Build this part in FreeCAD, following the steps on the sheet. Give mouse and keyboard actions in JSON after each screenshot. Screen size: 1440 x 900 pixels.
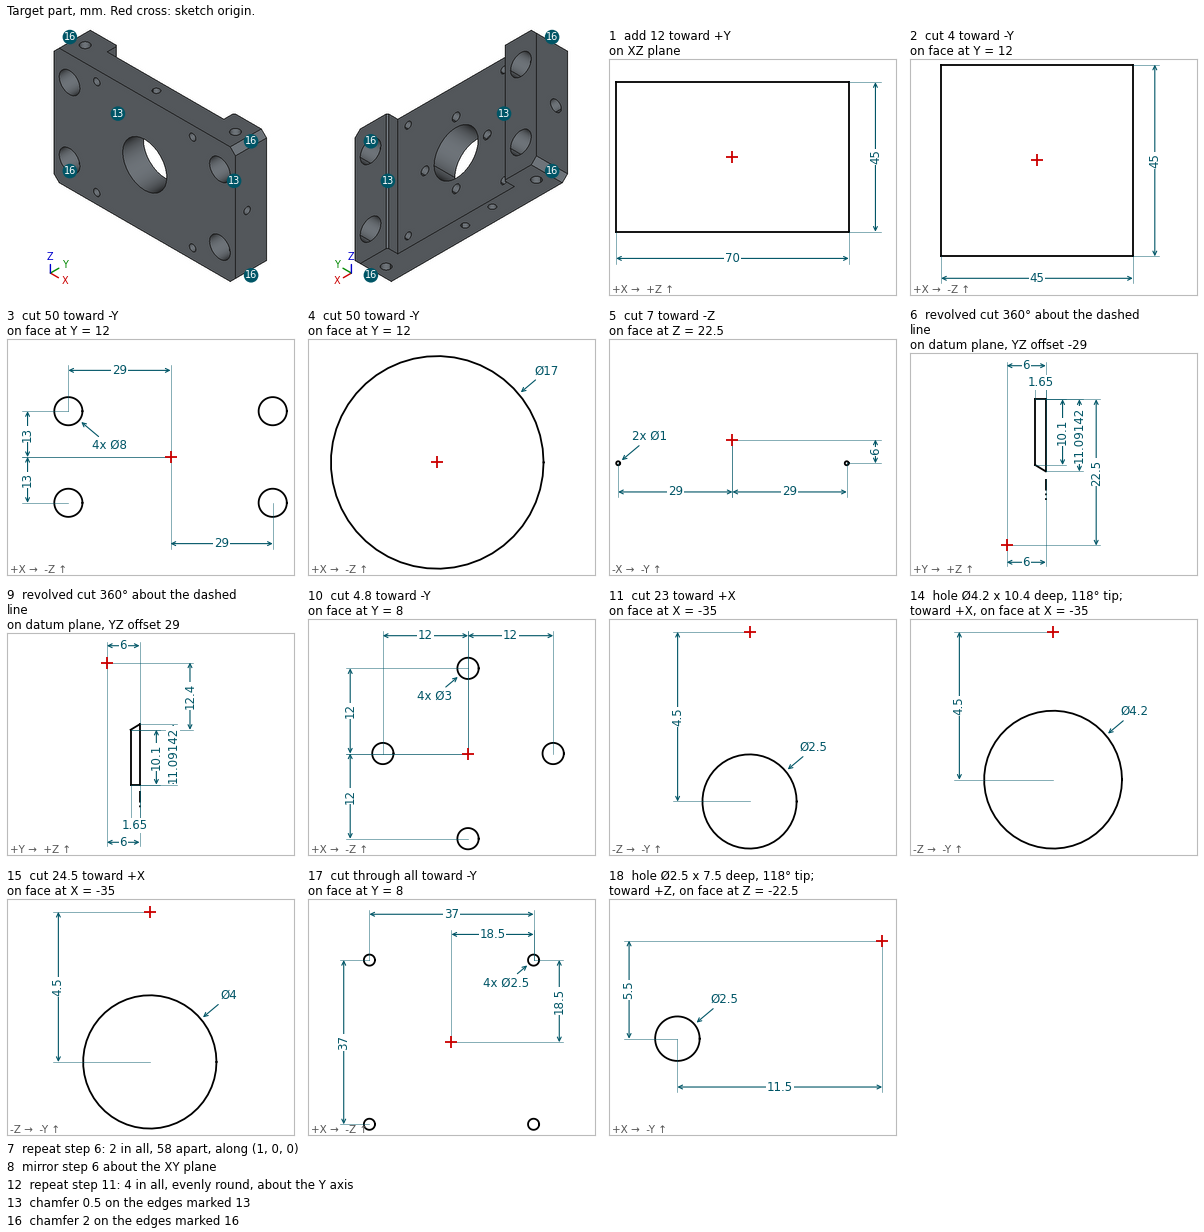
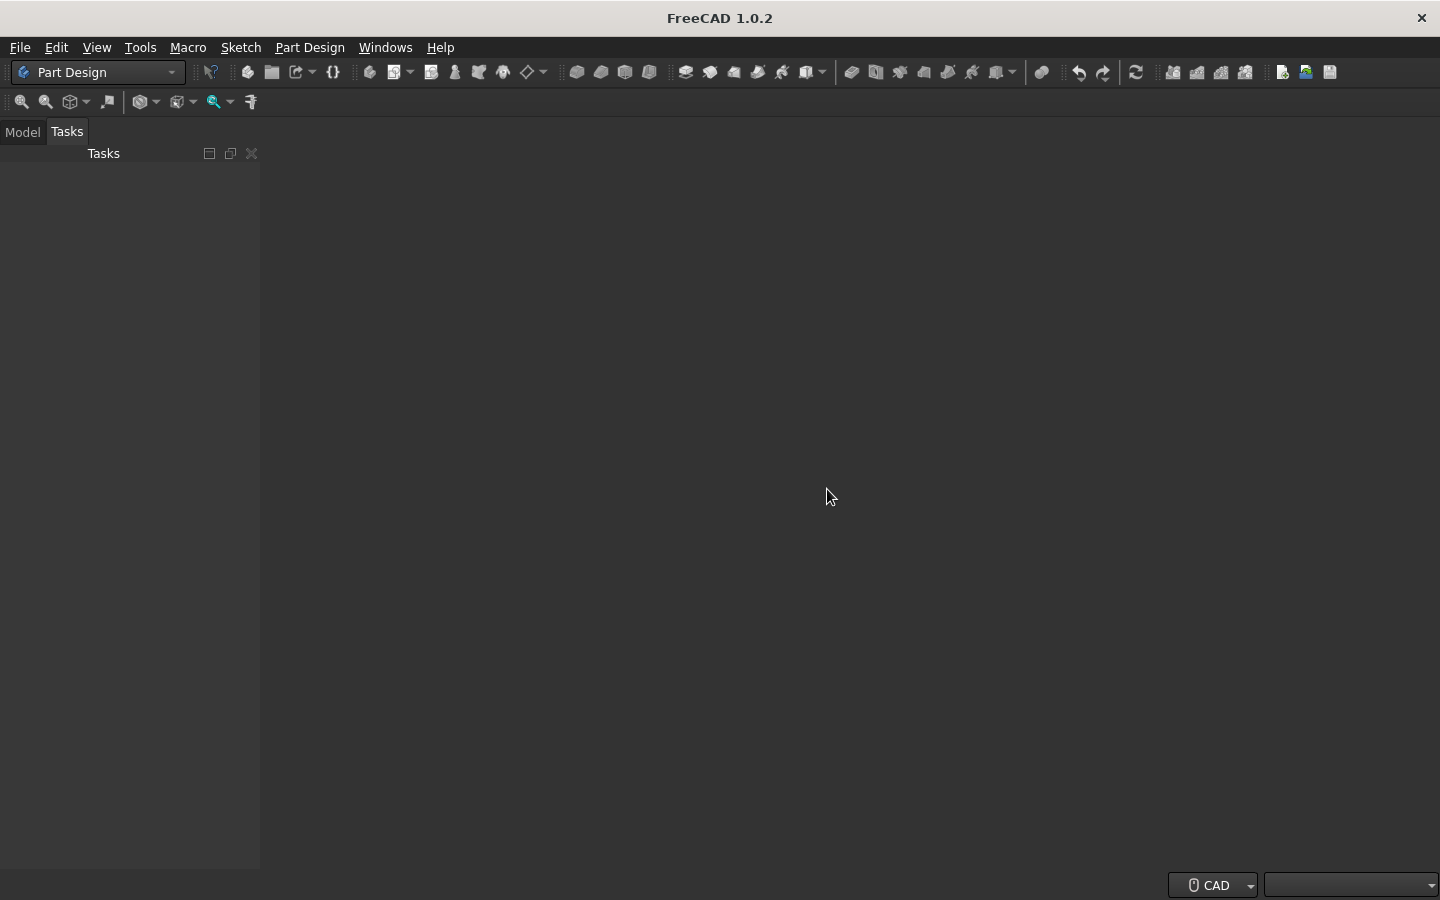
{"action": "left_click", "coordinate": [1282, 72]}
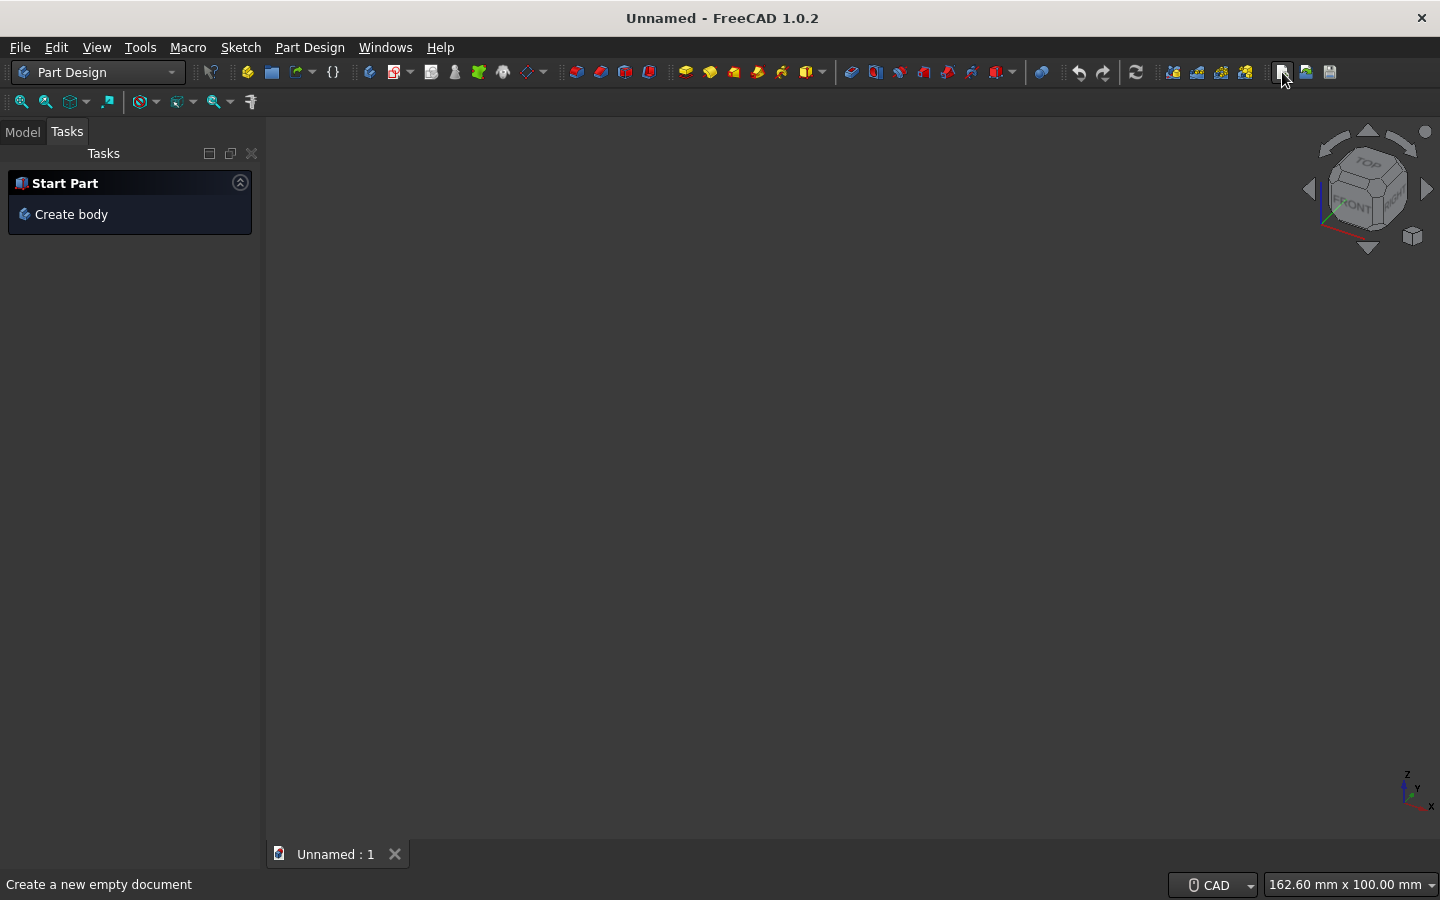
{"action": "left_click", "coordinate": [394, 72]}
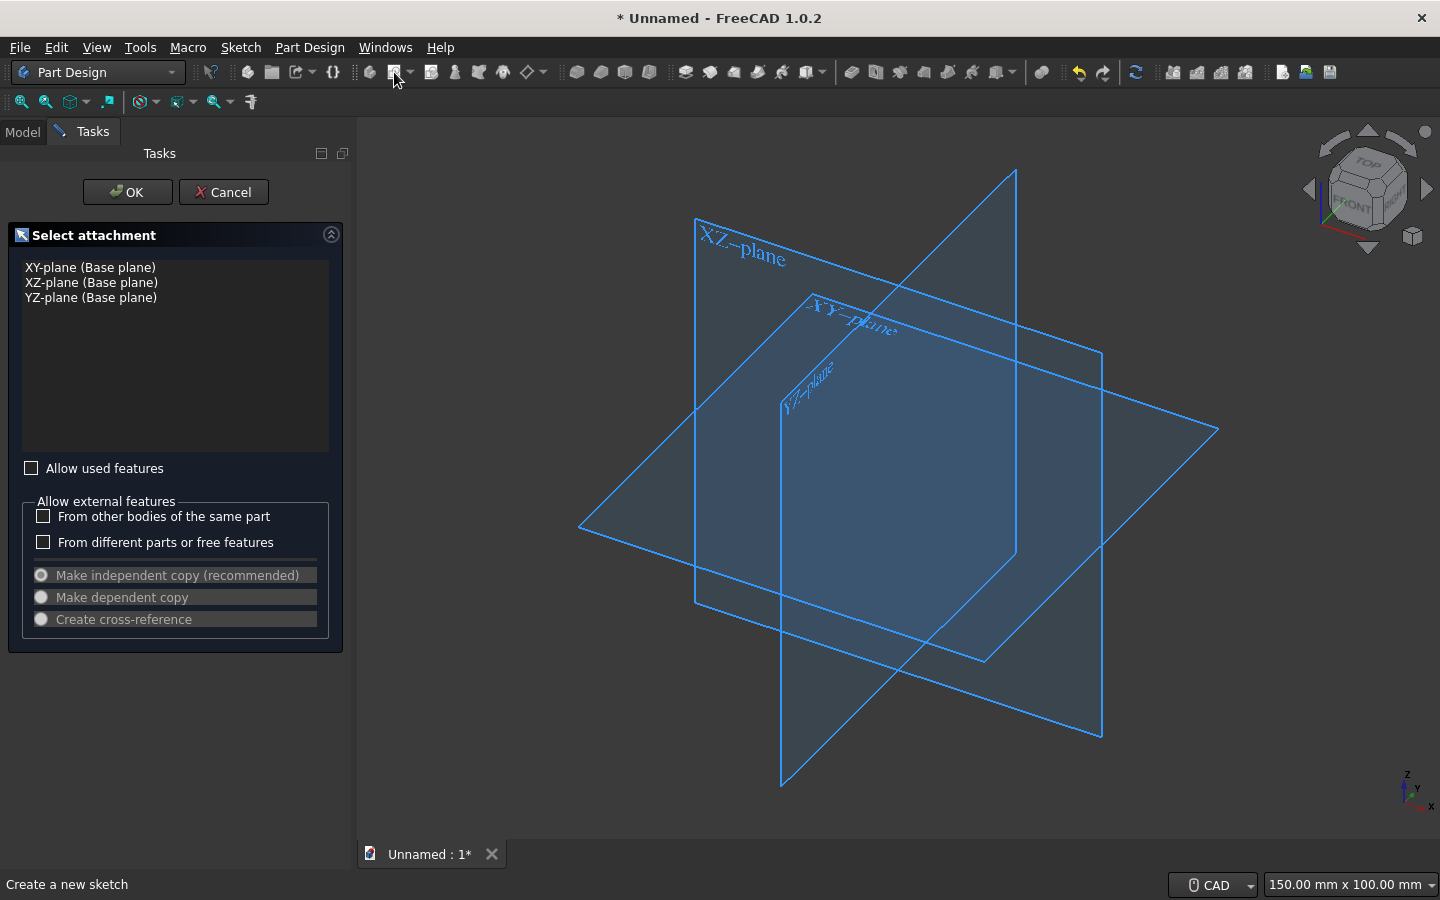
{"action": "left_click", "coordinate": [82, 282]}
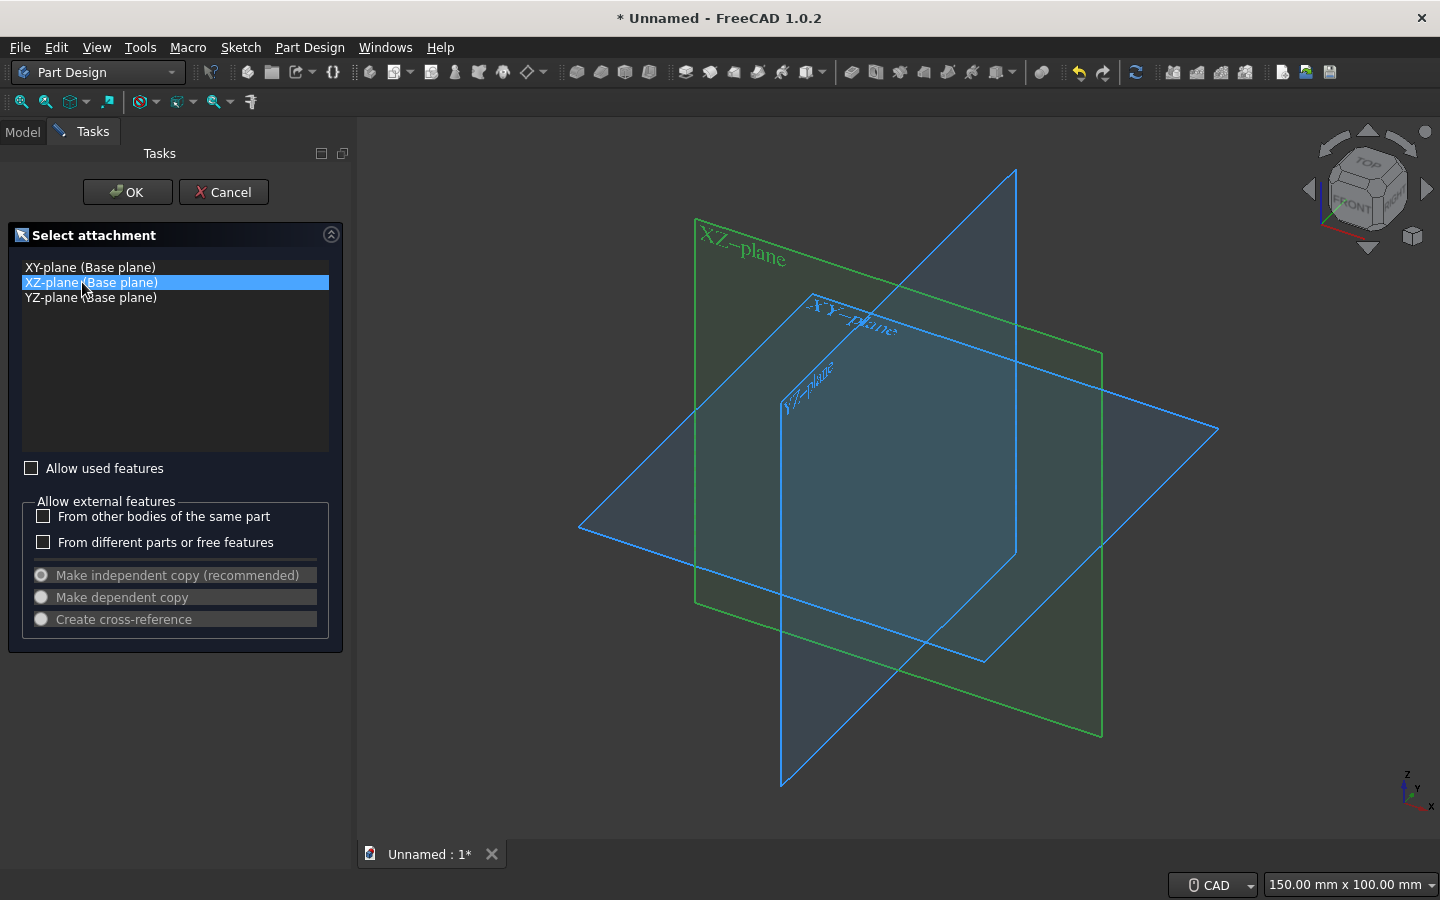
{"action": "left_click", "coordinate": [128, 192]}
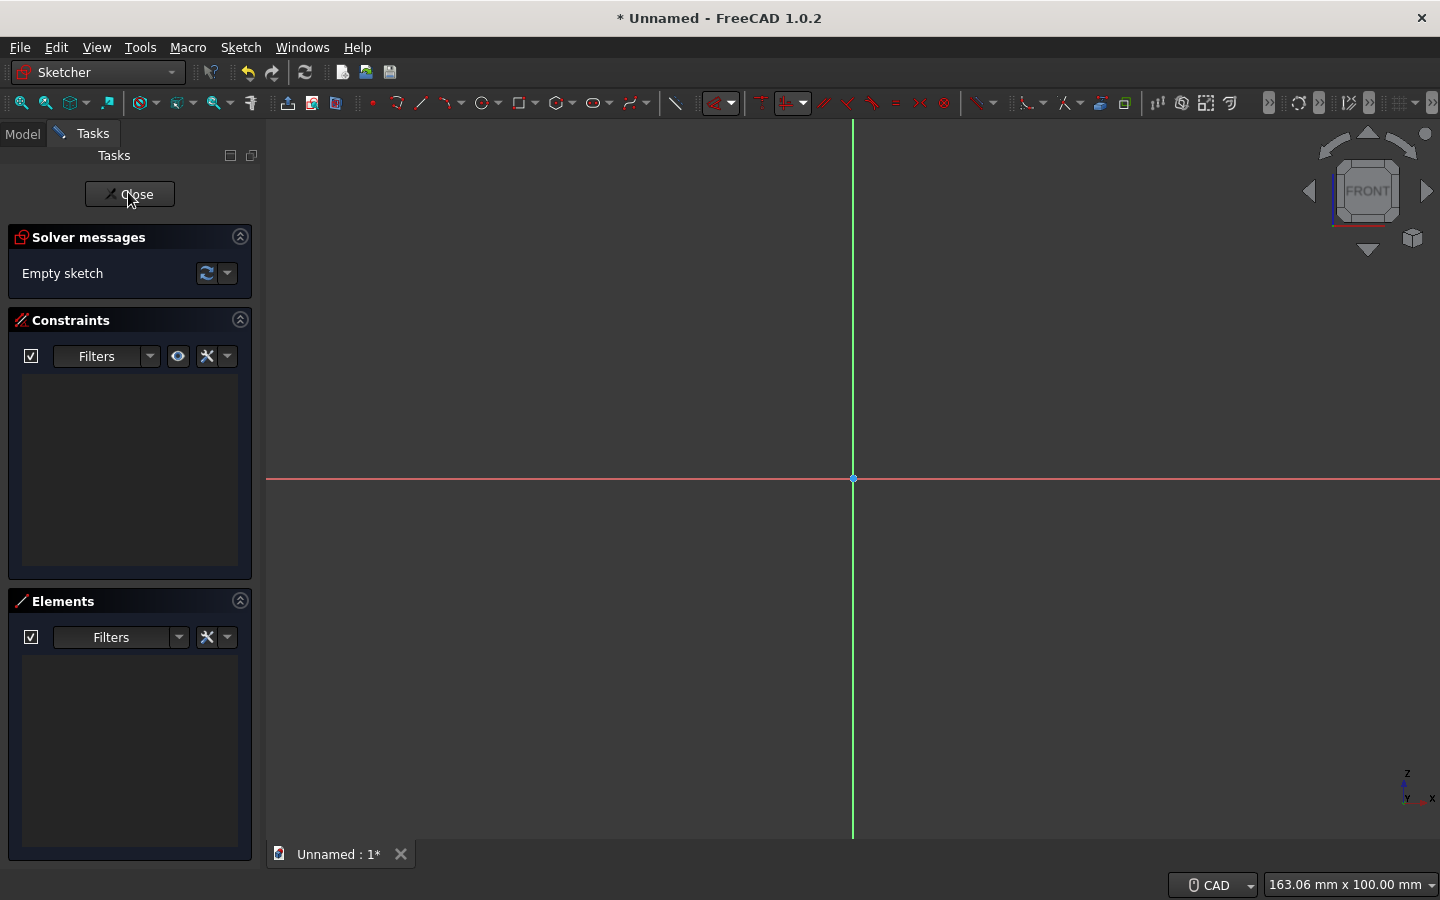
{"action": "scroll", "coordinate": [992, 479], "scroll_direction": "up", "scroll_amount": 2}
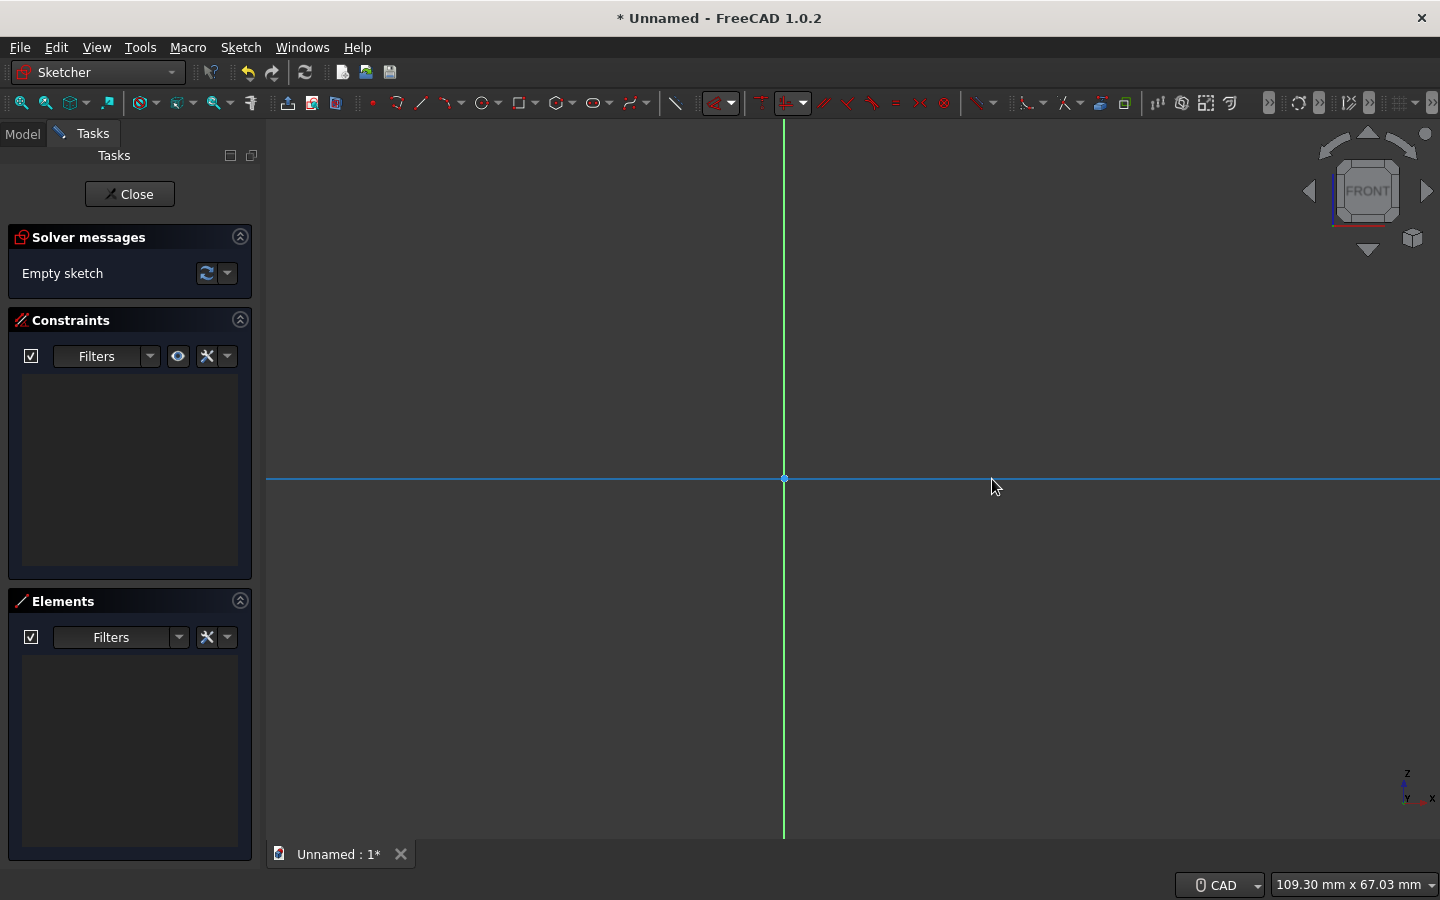
{"action": "key", "text": "g v"}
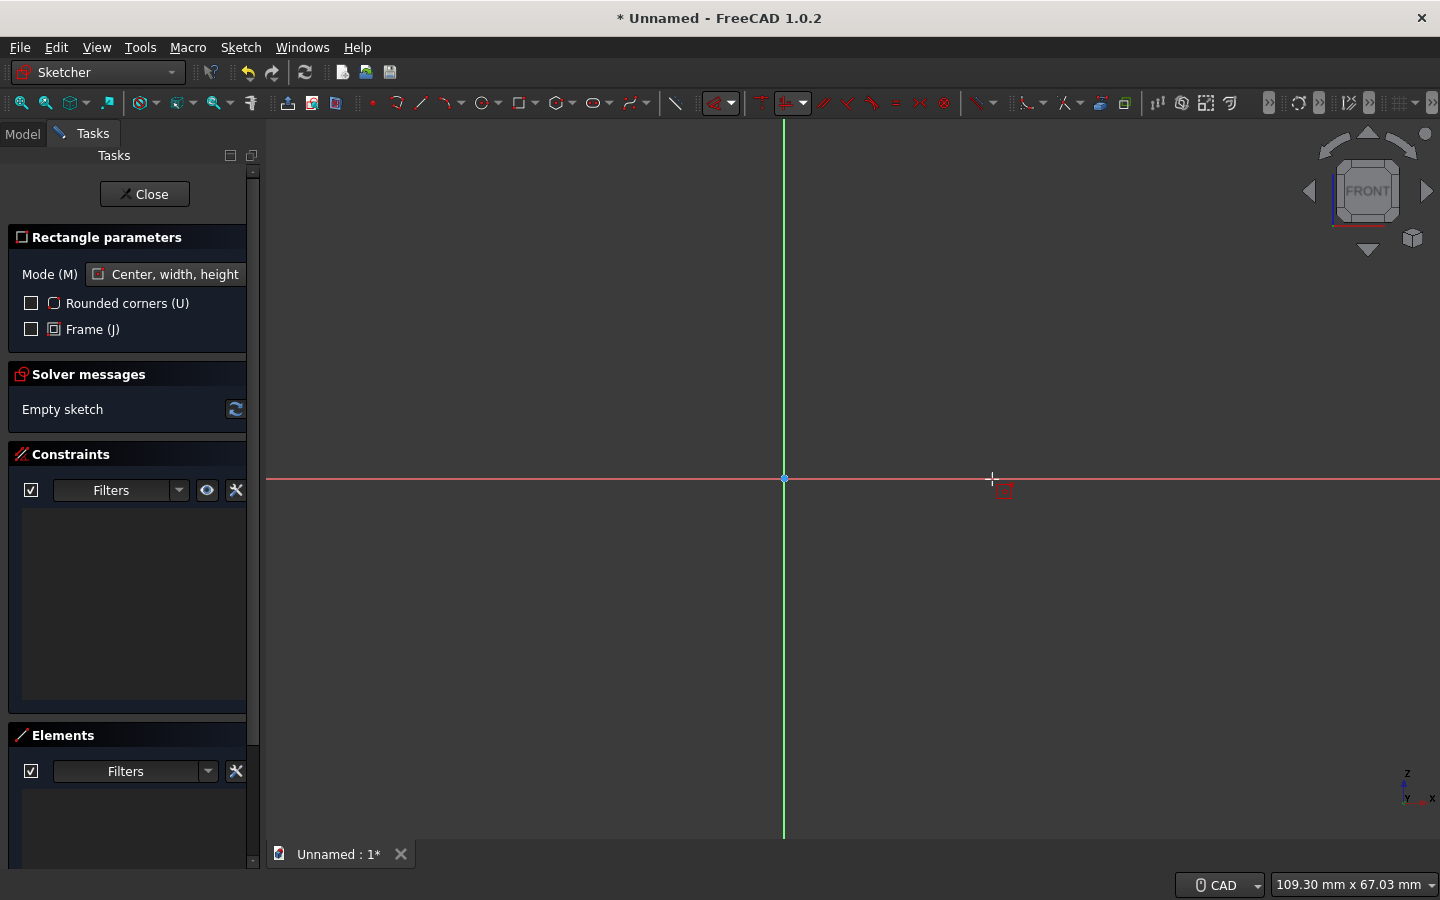
{"action": "left_click", "coordinate": [784, 479]}
{"action": "mouse_move", "coordinate": [1160, 237]}